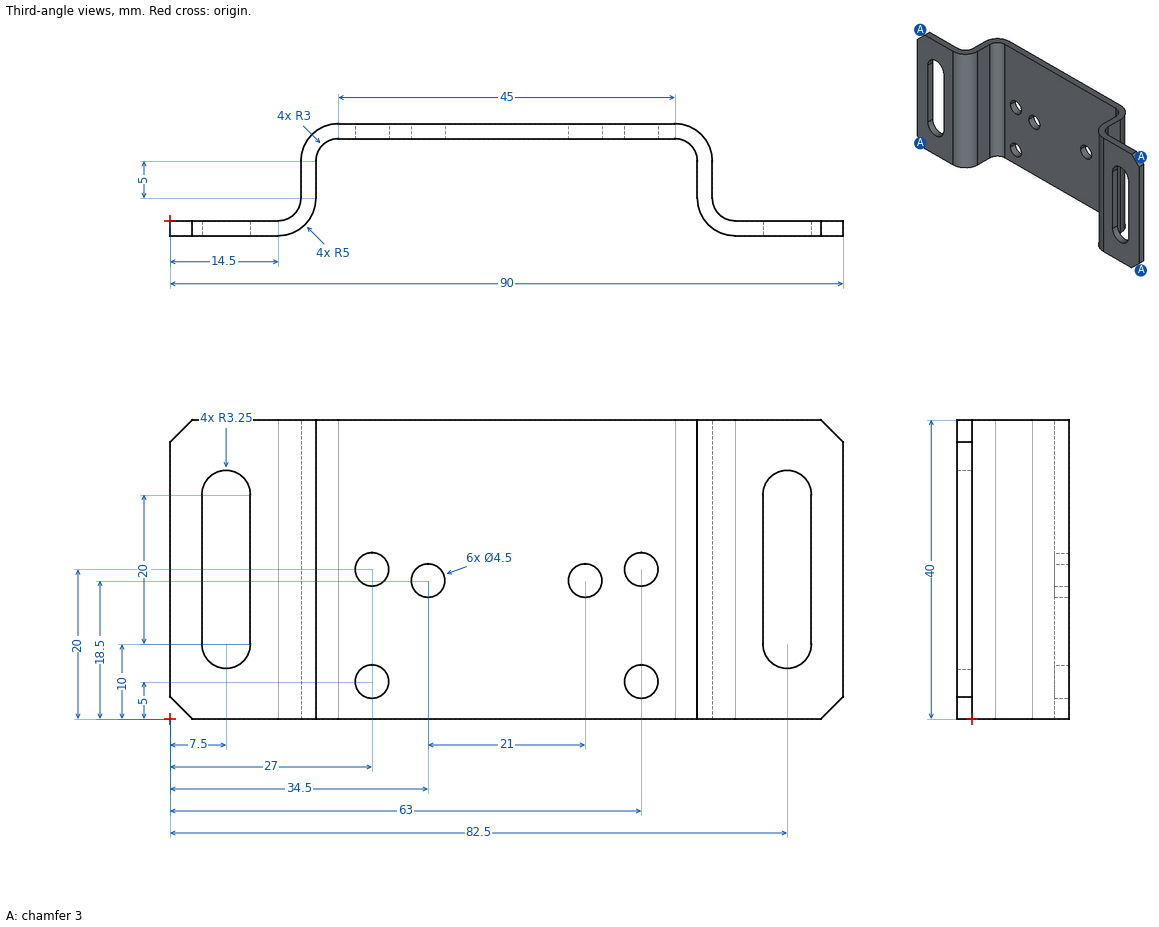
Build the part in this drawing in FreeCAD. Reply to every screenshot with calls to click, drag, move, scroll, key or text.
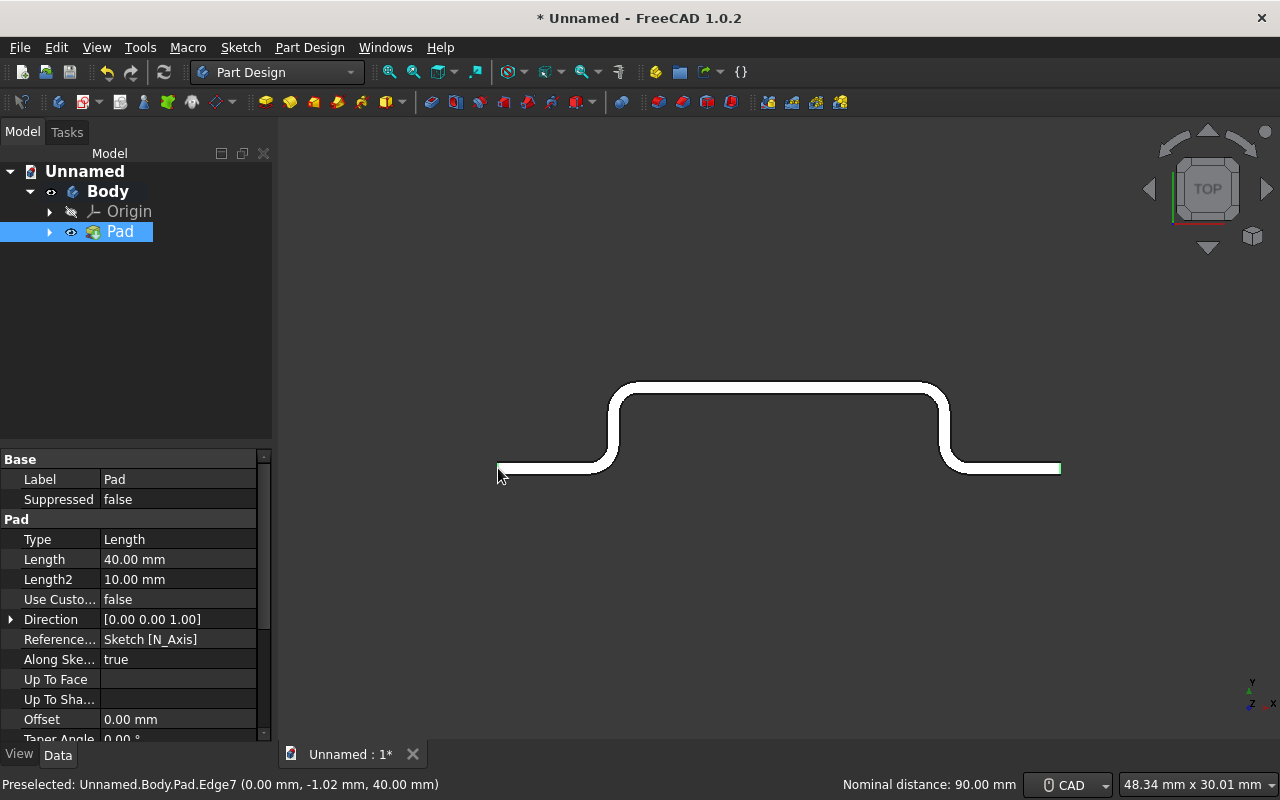
key(1)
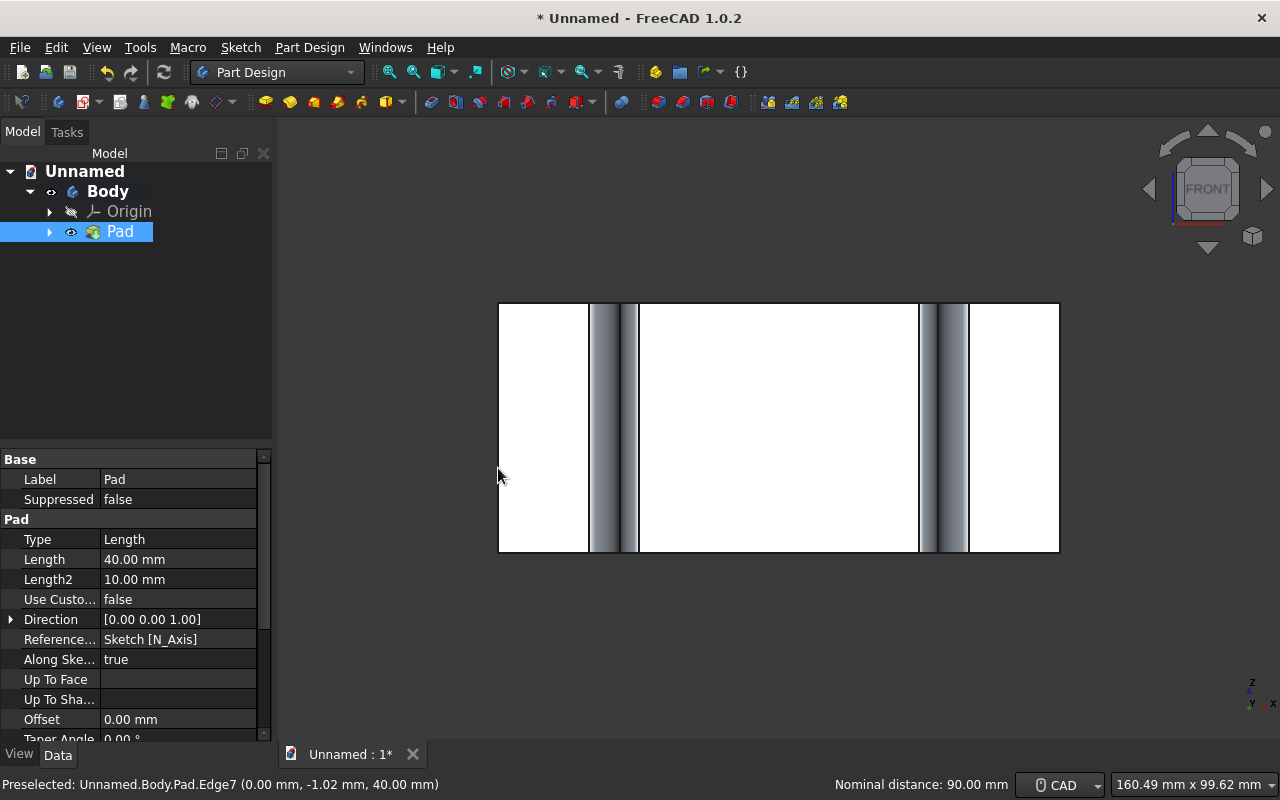
scroll(498, 552, up, 6)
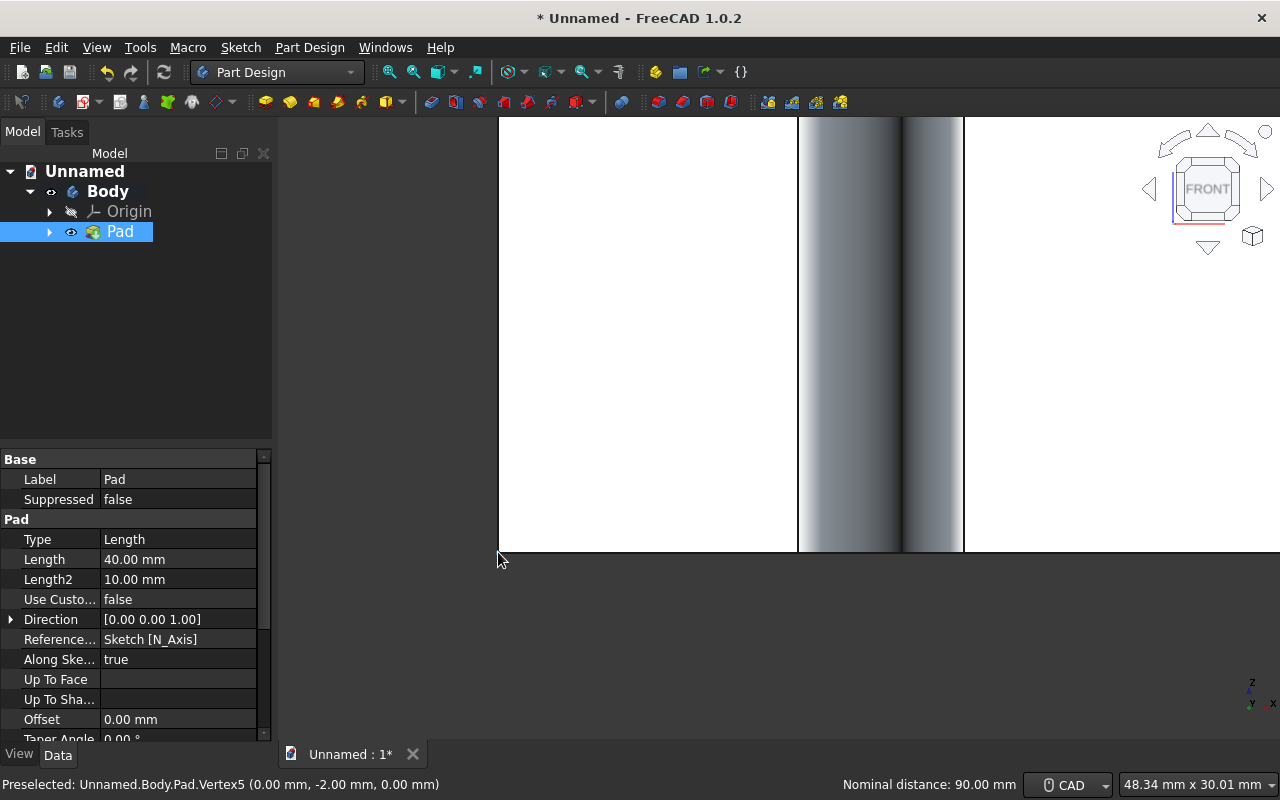
click(390, 72)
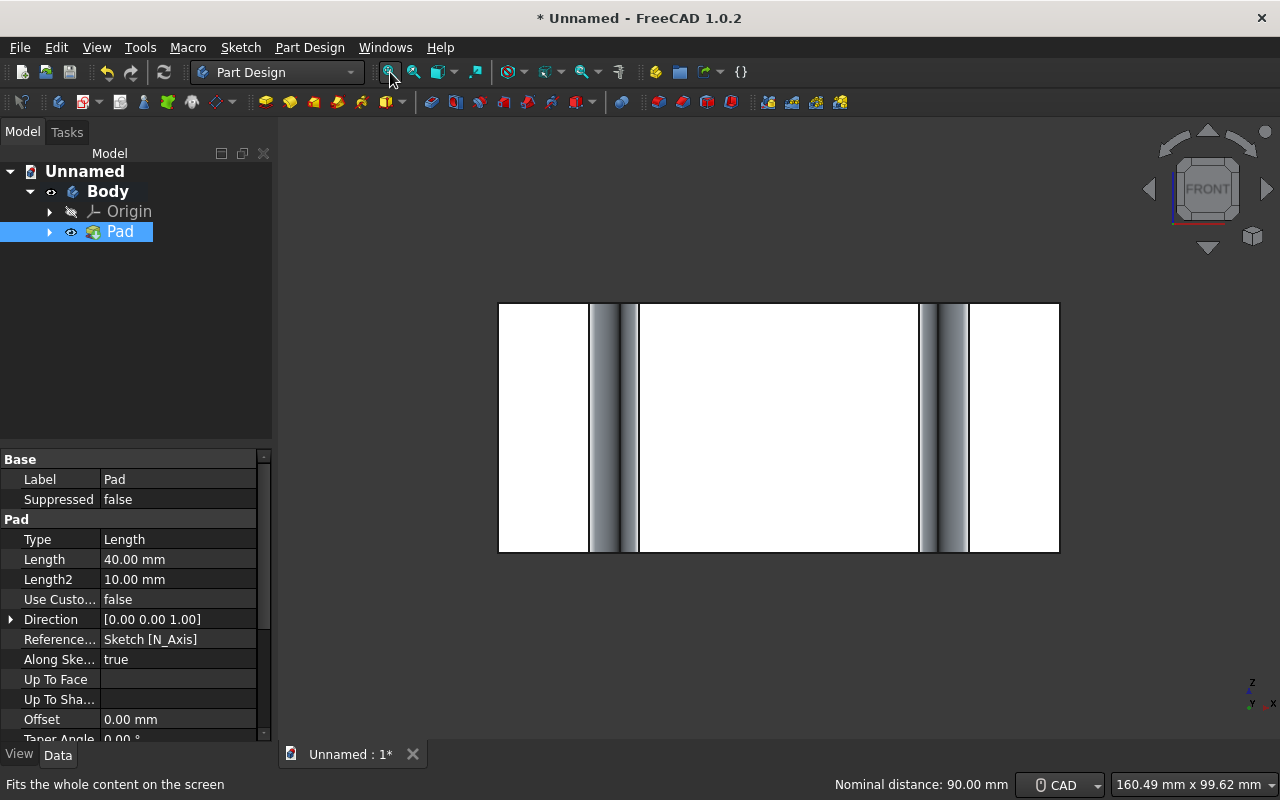
key(3)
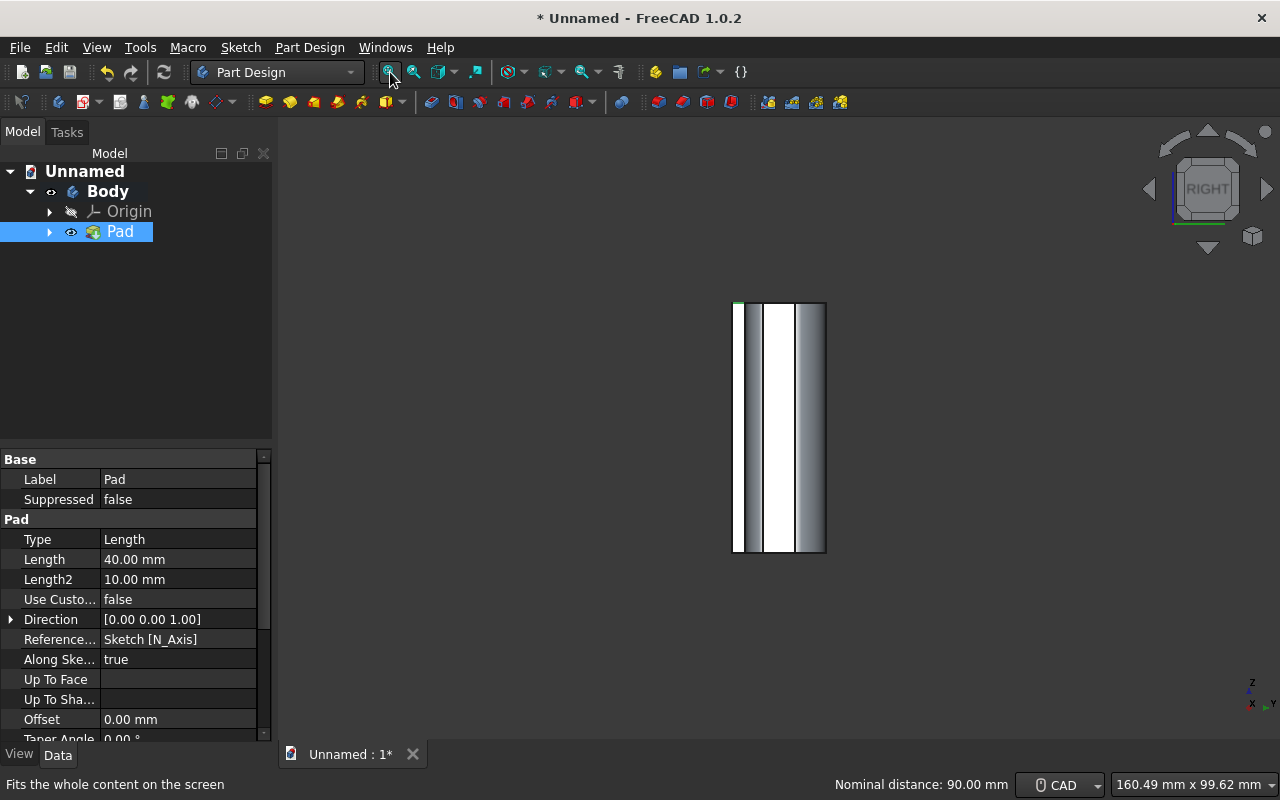
key(v)
key(f)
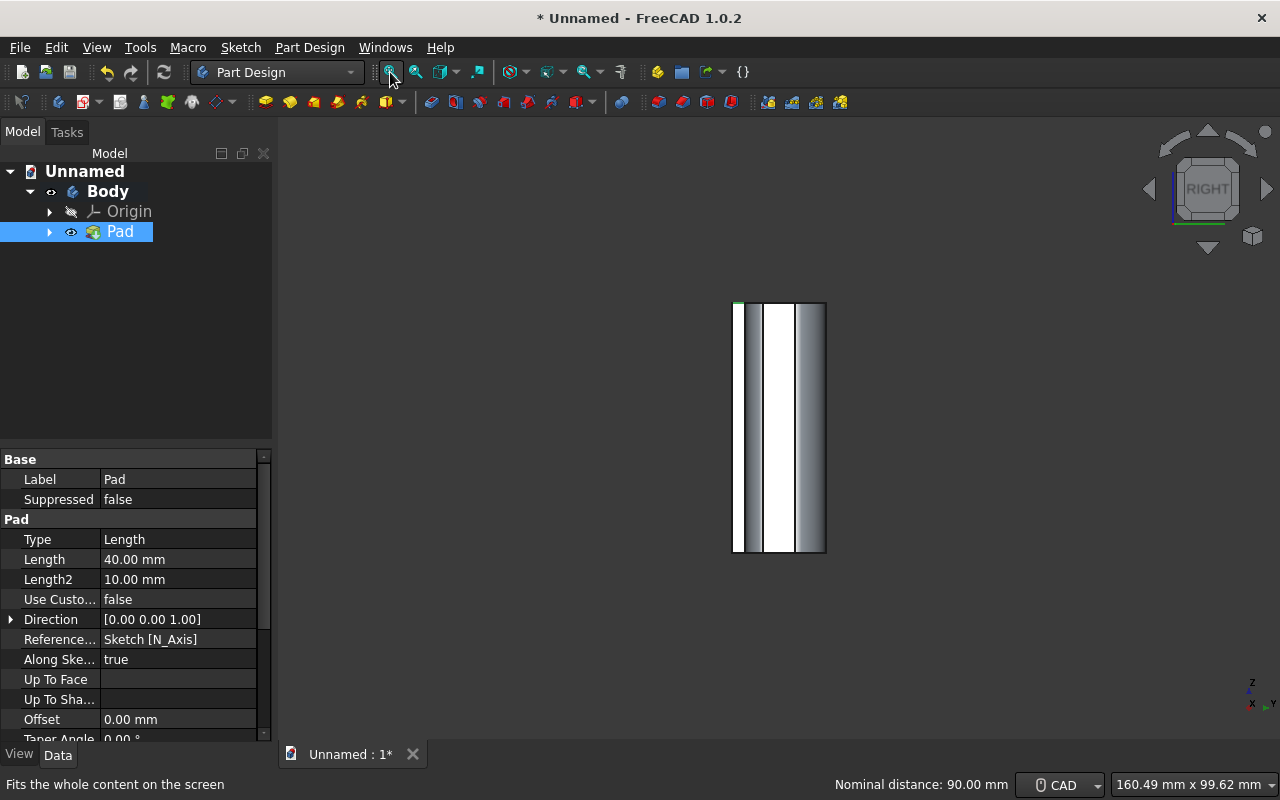
scroll(738, 552, up, 6)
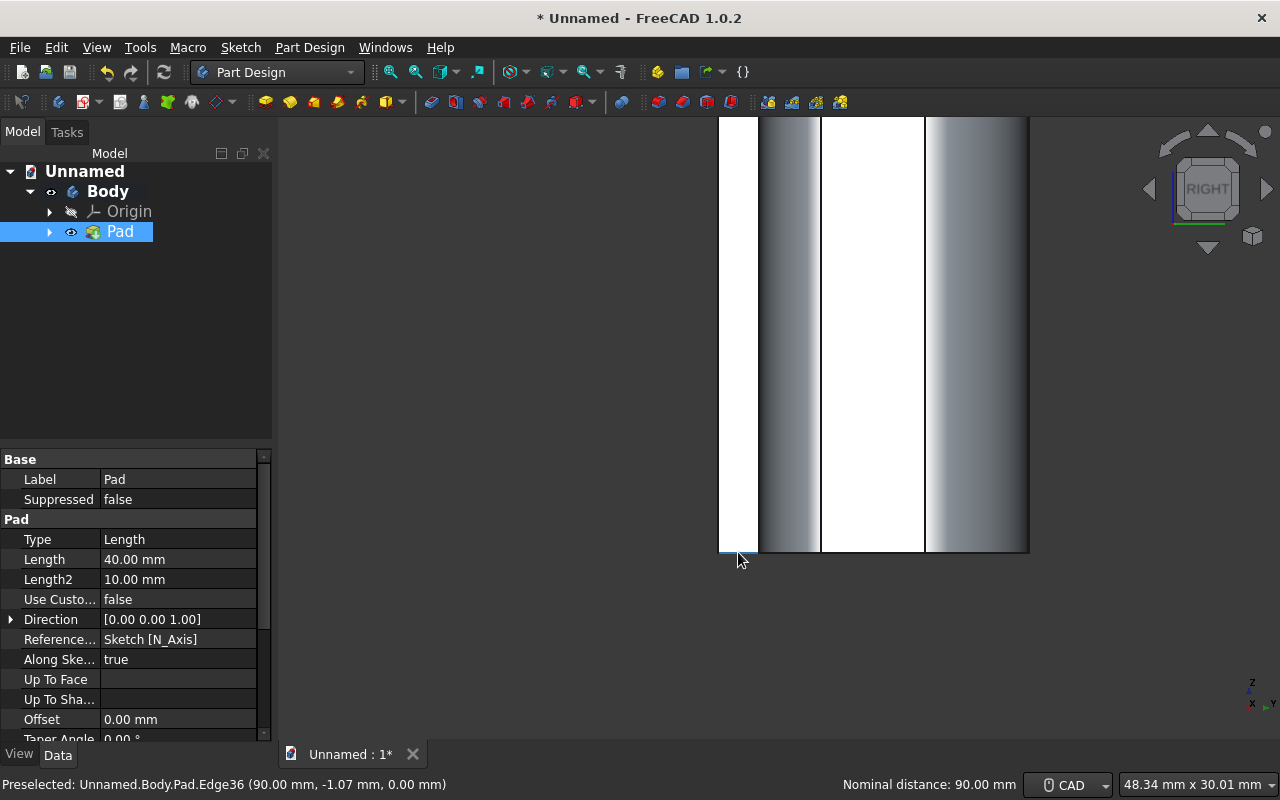
click(738, 552, ctrl)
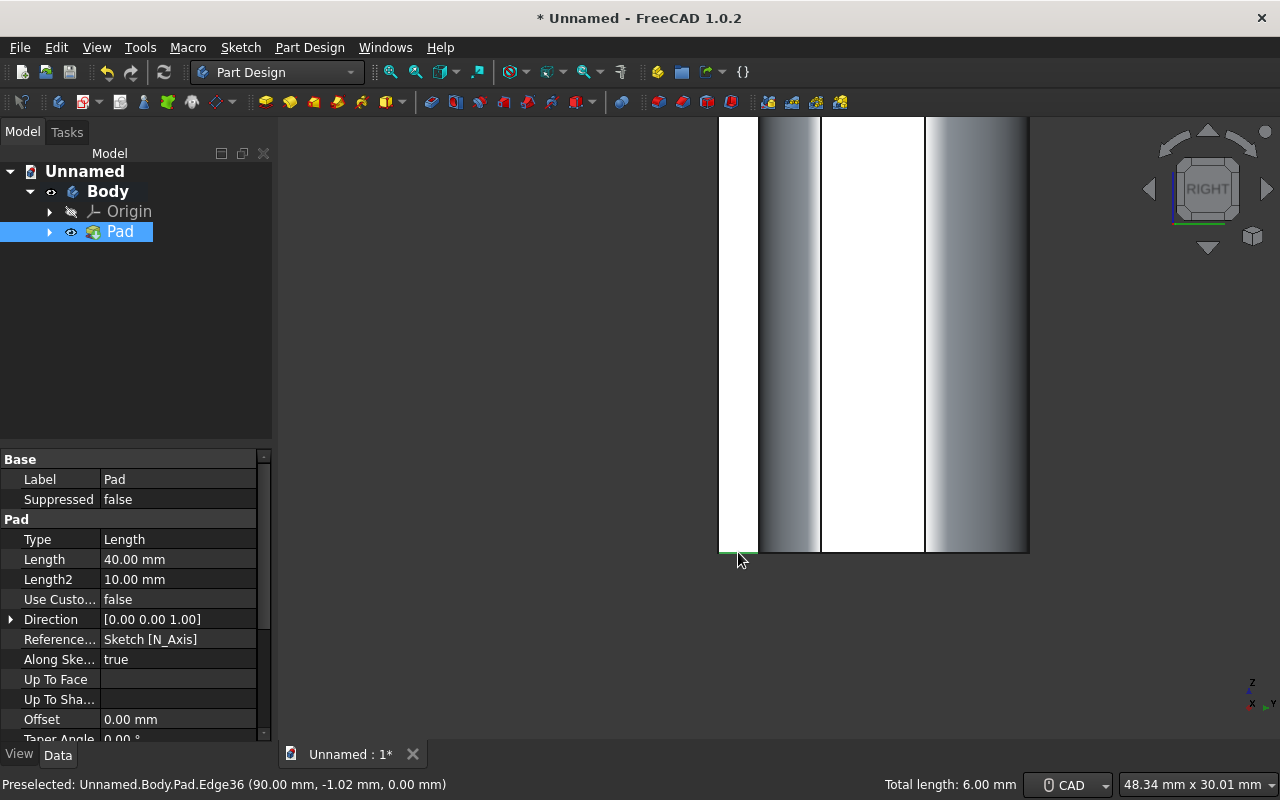
key(v)
key(f)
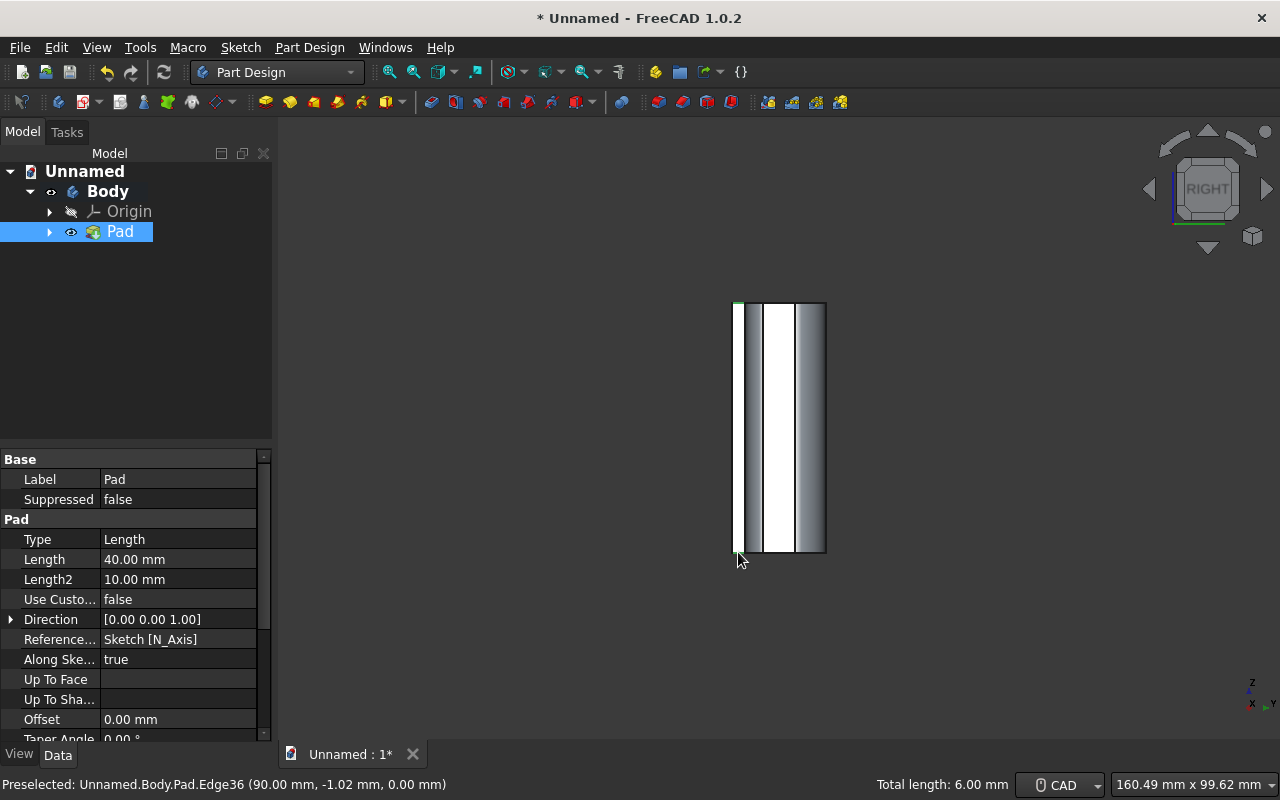
key(5)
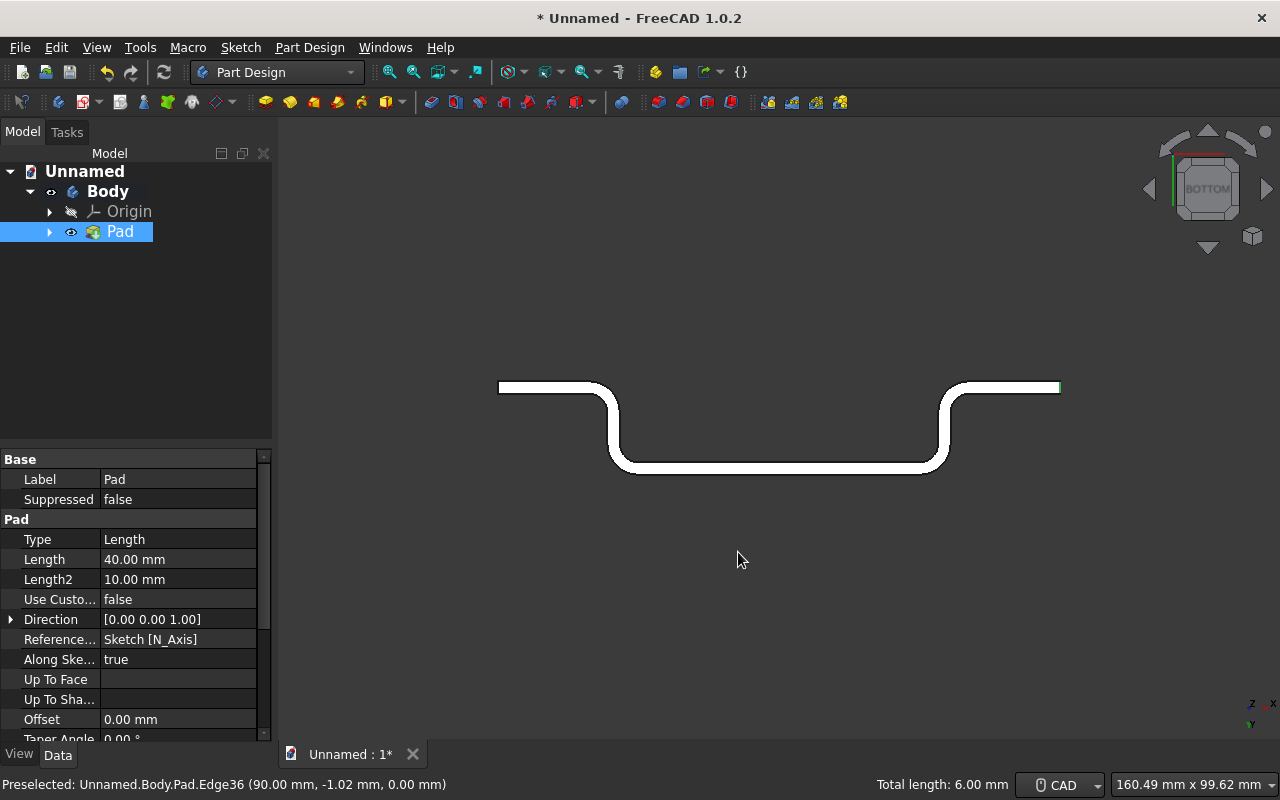
scroll(498, 386, up, 6)